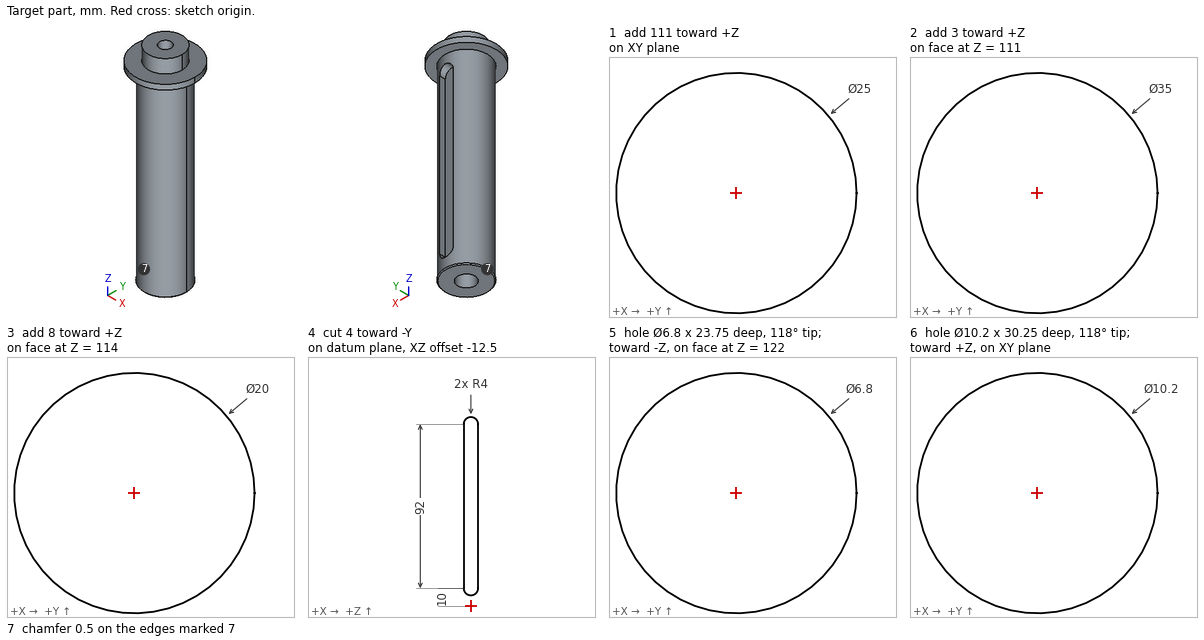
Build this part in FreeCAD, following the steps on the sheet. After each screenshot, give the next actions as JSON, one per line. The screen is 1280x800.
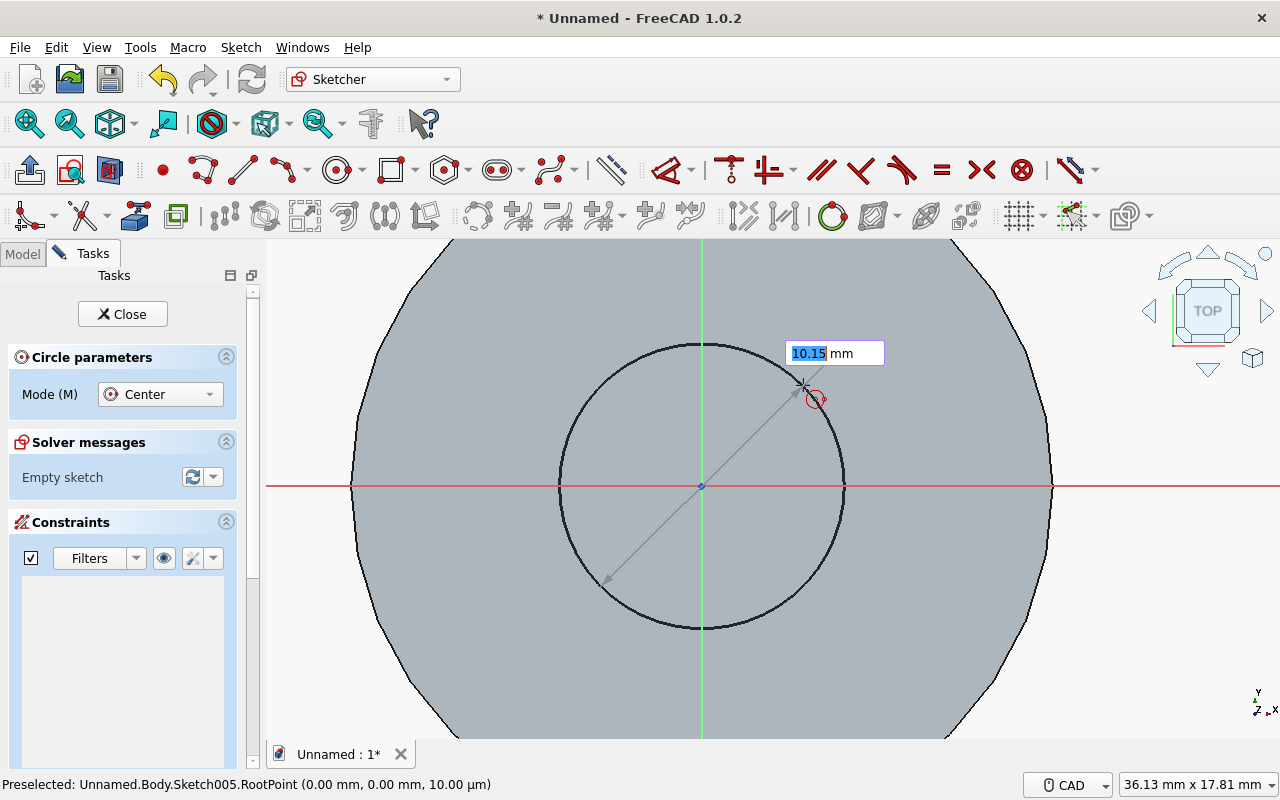
{"action": "type", "text": "10.2"}
{"action": "key", "text": "Return"}
{"action": "key", "text": "Escape"}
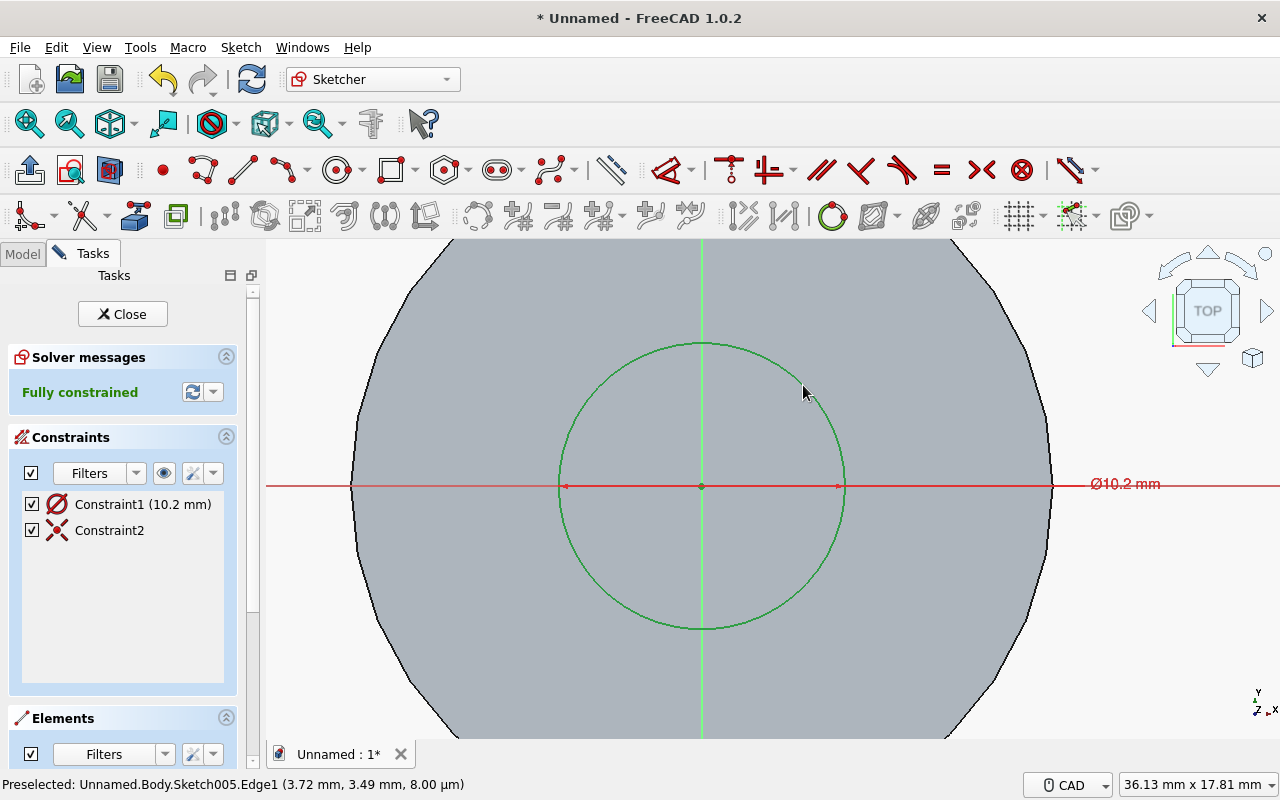
{"action": "left_click", "coordinate": [123, 314]}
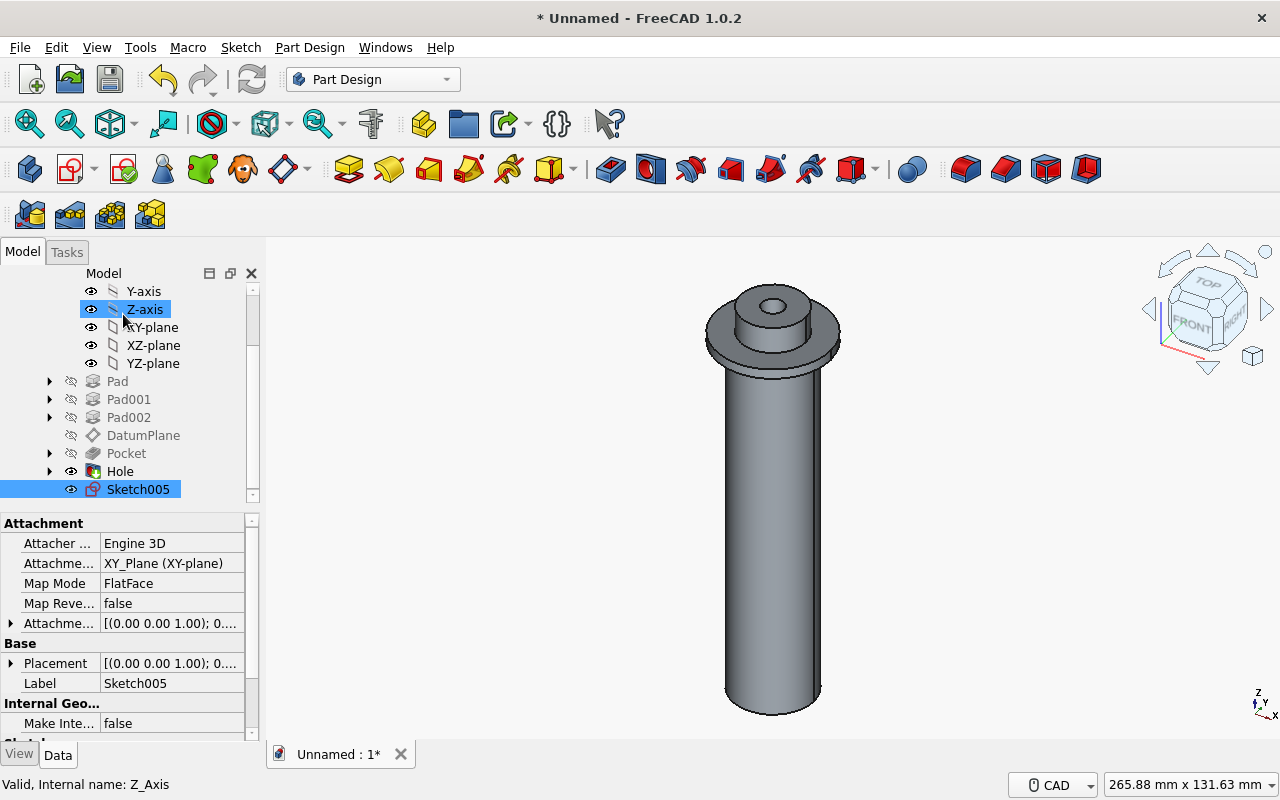
{"action": "left_click", "coordinate": [652, 170]}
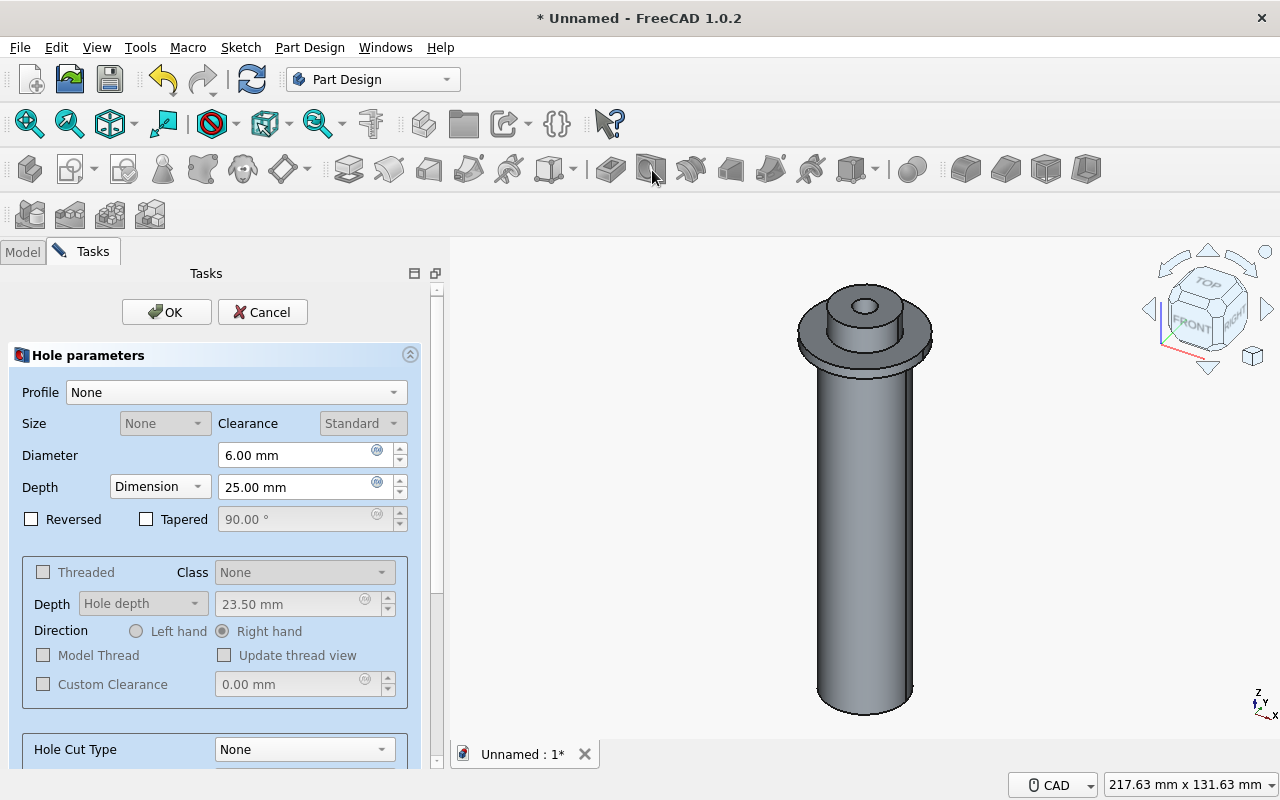
{"action": "triple_click", "coordinate": [305, 455]}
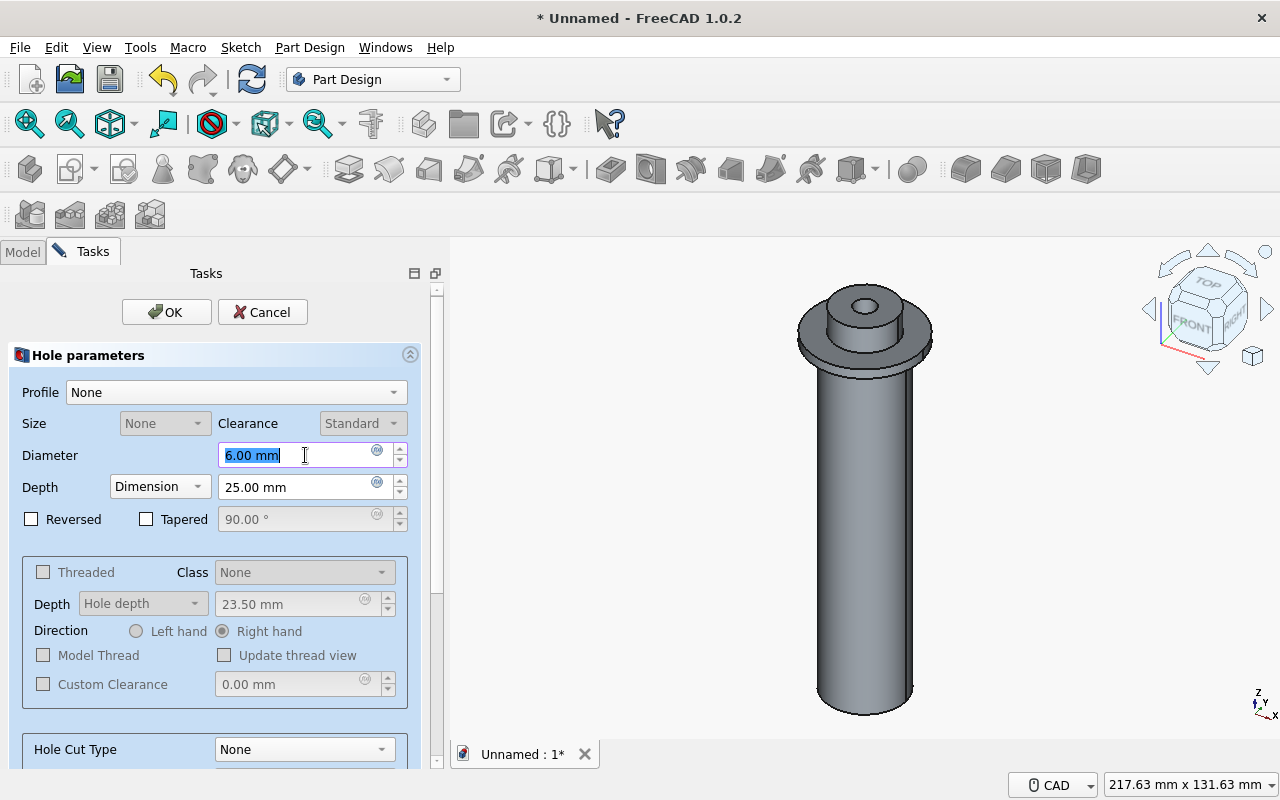
{"action": "type", "text": "10.2"}
{"action": "key", "text": "Tab"}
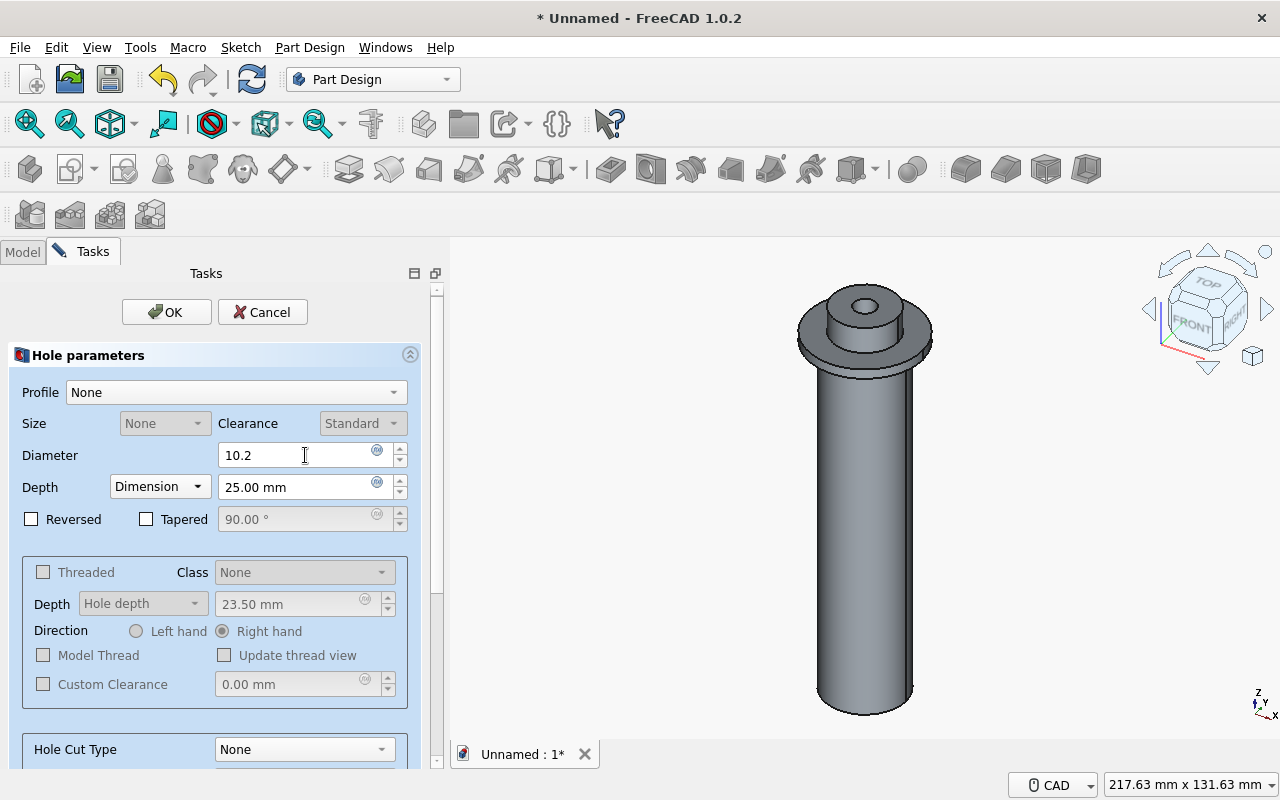
{"action": "triple_click", "coordinate": [305, 487]}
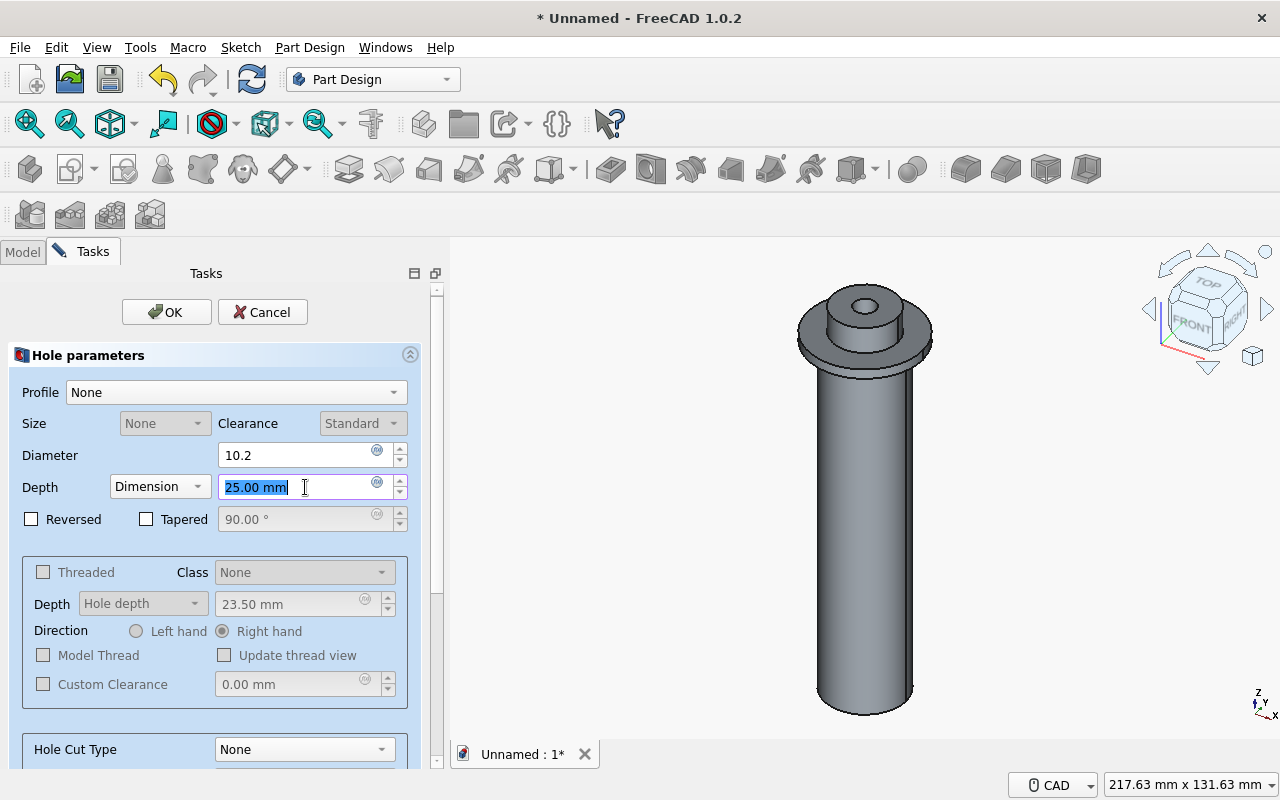
{"action": "type", "text": "30.25"}
{"action": "key", "text": "Tab"}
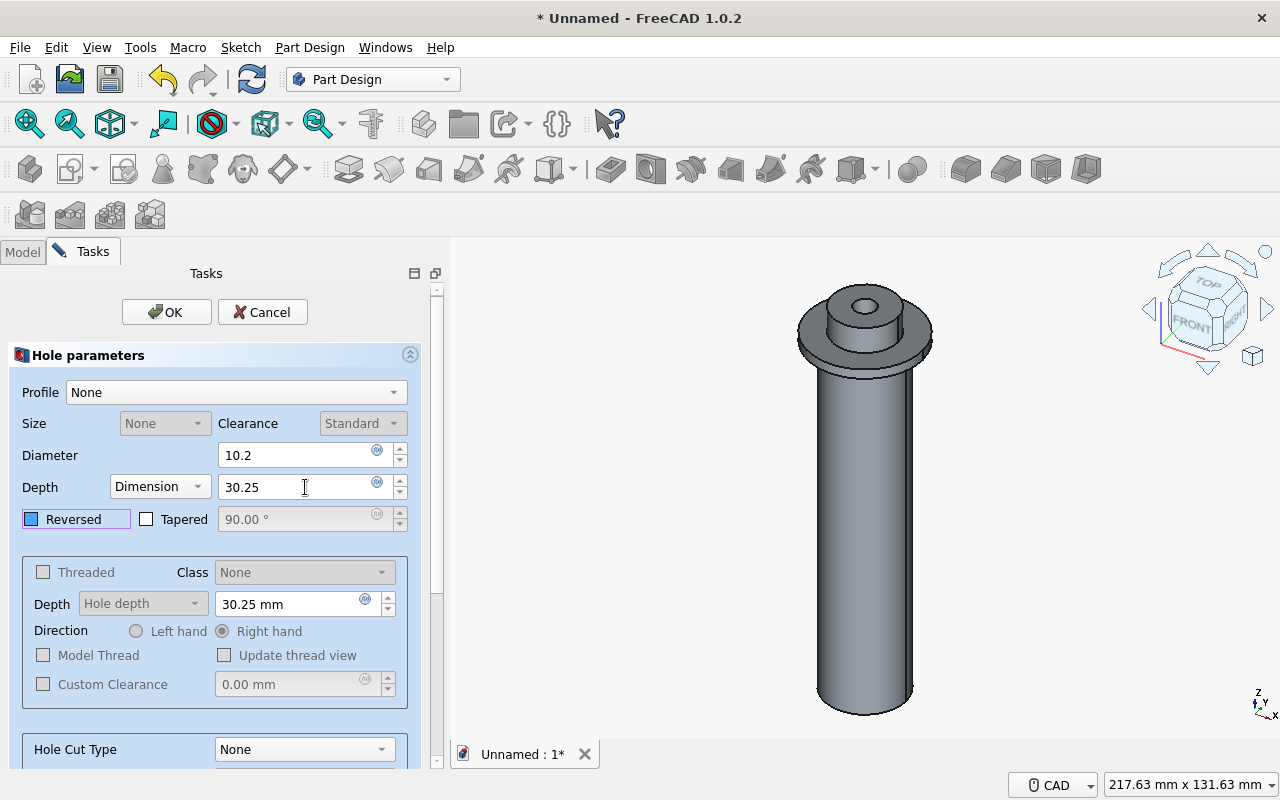
{"action": "left_click", "coordinate": [30, 519]}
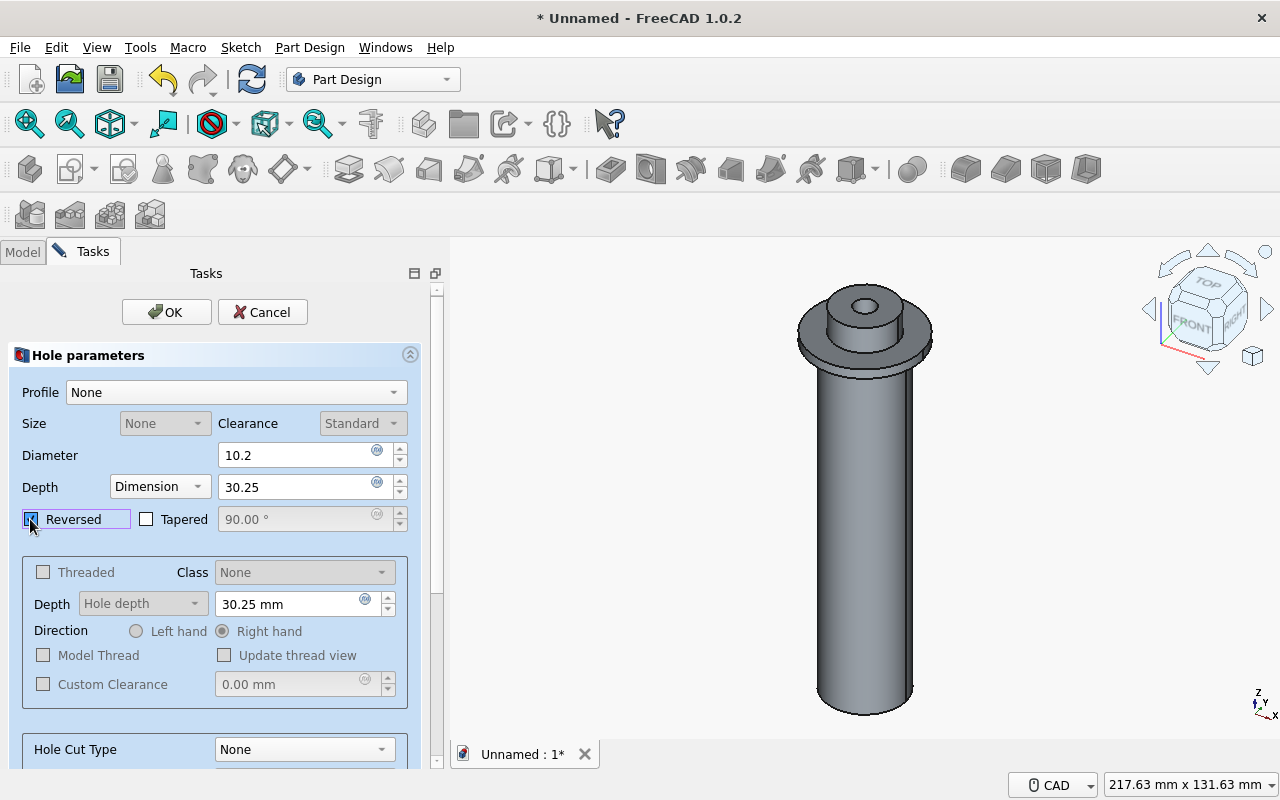
{"action": "left_click", "coordinate": [167, 312]}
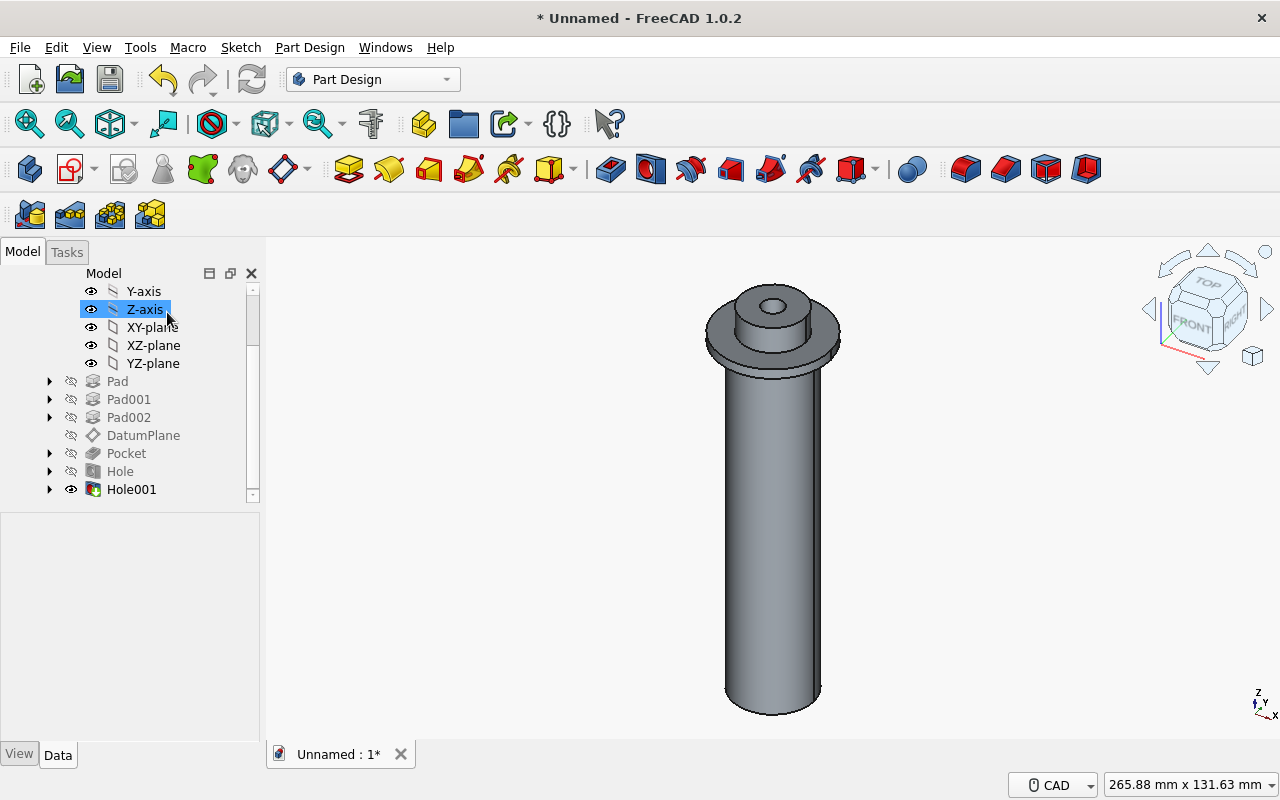
{"action": "key", "text": "0"}